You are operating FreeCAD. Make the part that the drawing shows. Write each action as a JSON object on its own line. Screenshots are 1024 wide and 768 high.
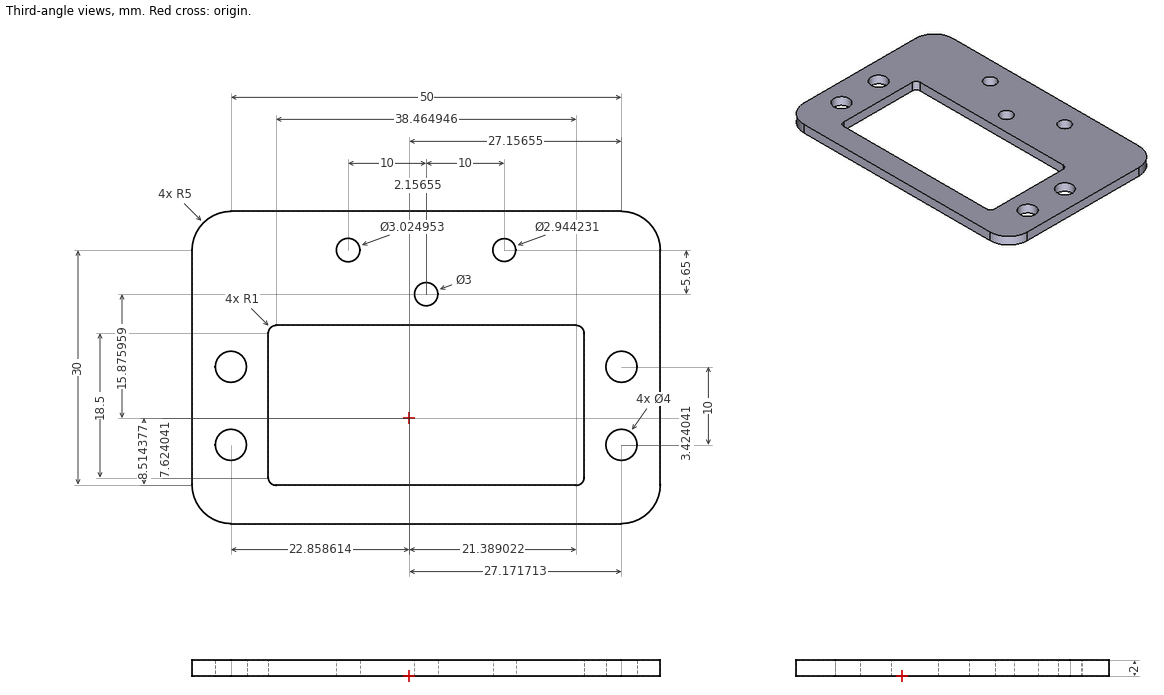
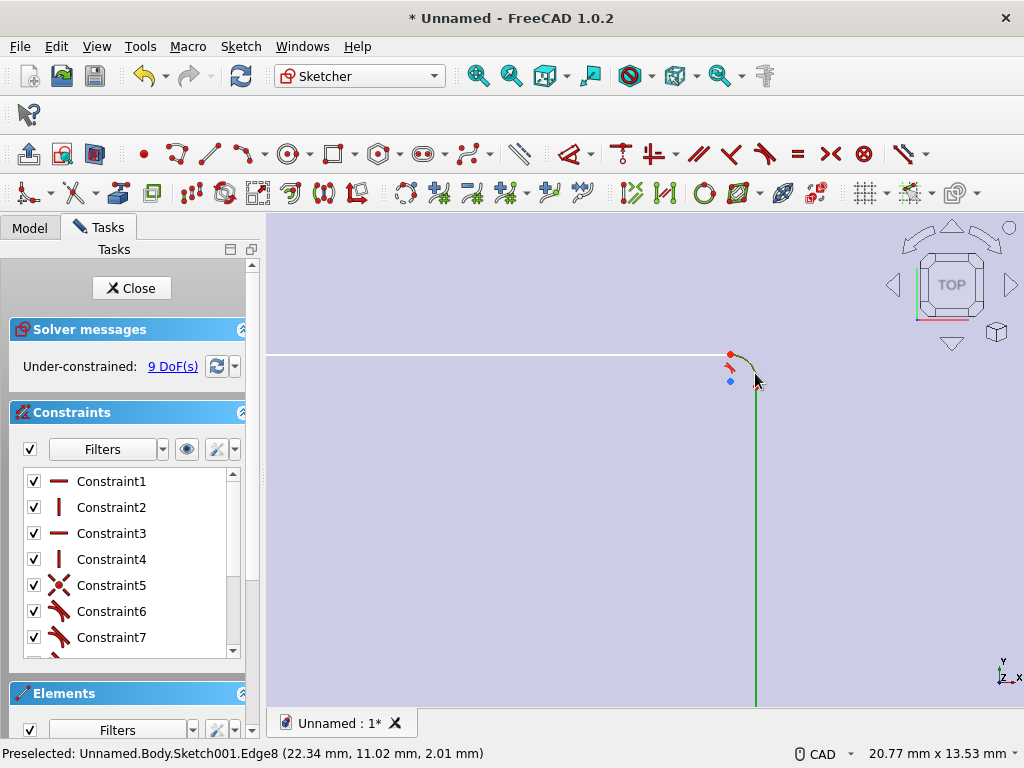
{"action": "key", "text": "t"}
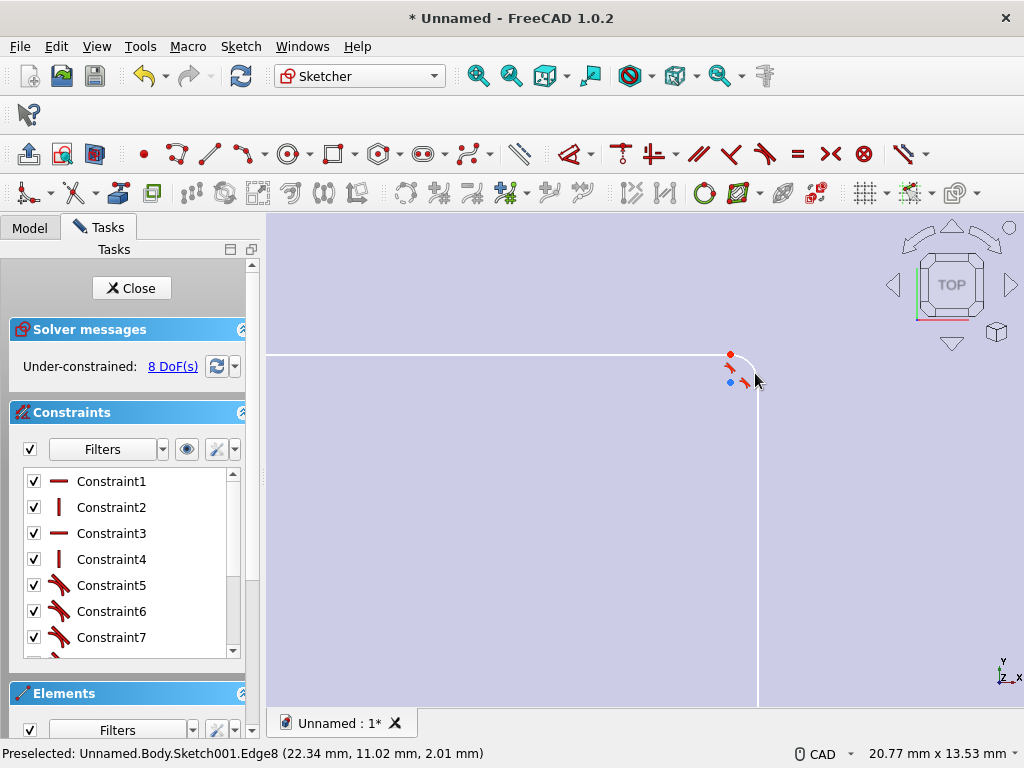
{"action": "scroll", "coordinate": [759, 375], "scroll_direction": "down", "scroll_amount": 7}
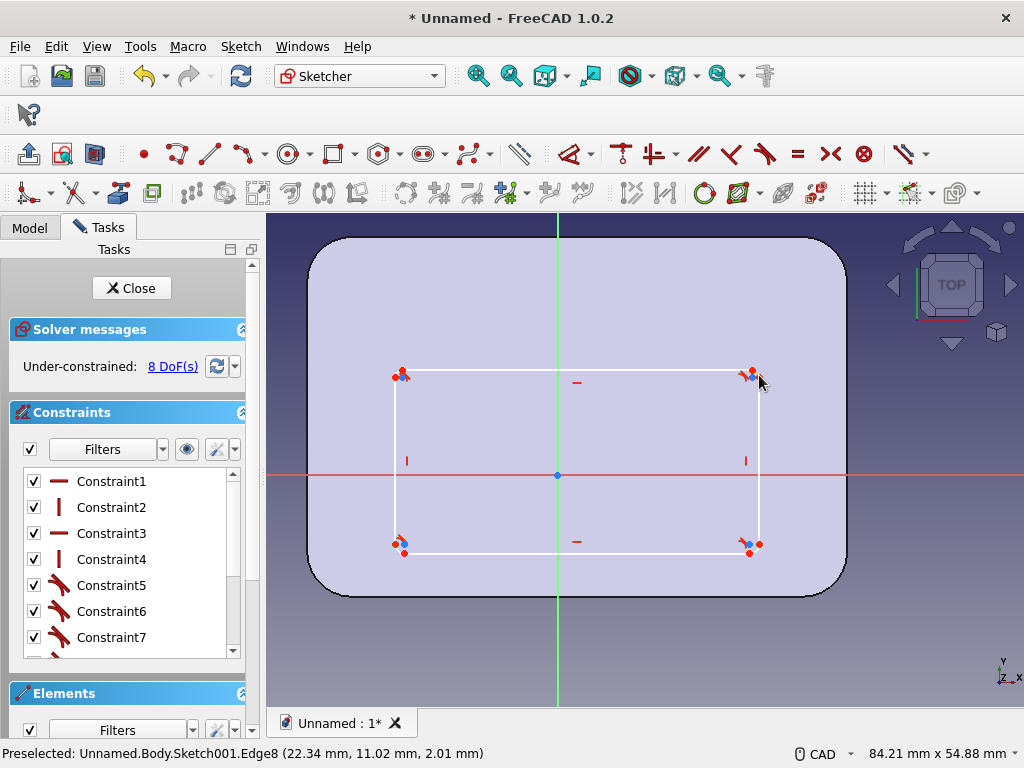
{"action": "scroll", "coordinate": [399, 371], "scroll_direction": "up", "scroll_amount": 7}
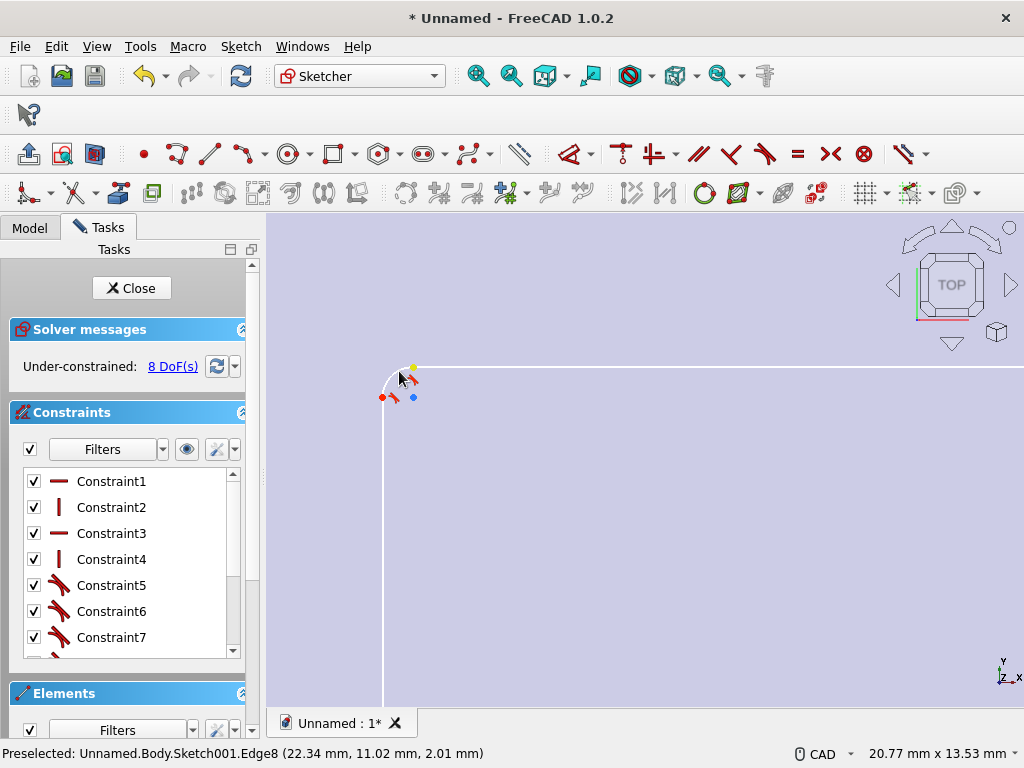
{"action": "left_click", "coordinate": [399, 370]}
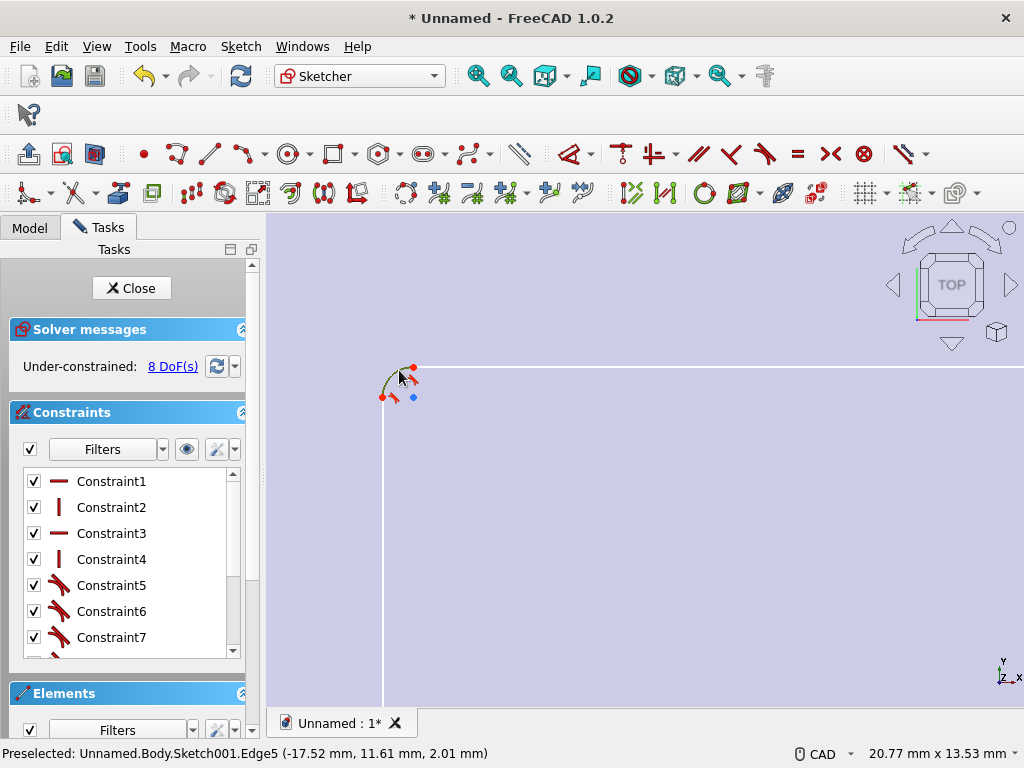
{"action": "scroll", "coordinate": [398, 371], "scroll_direction": "down", "scroll_amount": 7}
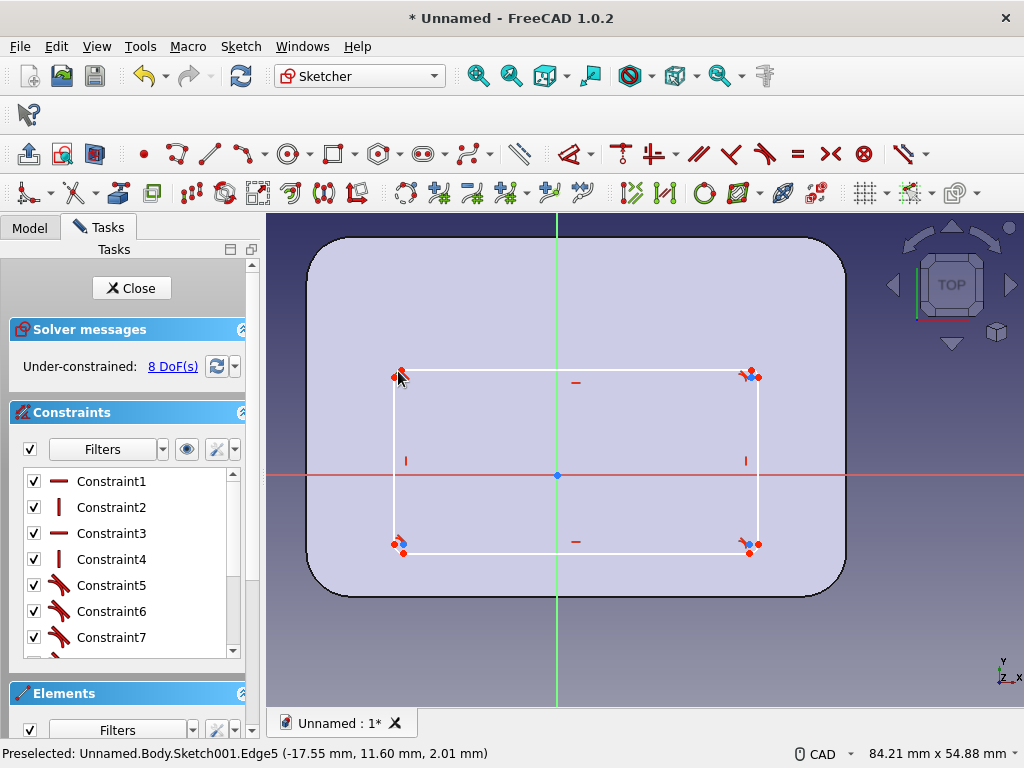
{"action": "scroll", "coordinate": [395, 548], "scroll_direction": "up", "scroll_amount": 6}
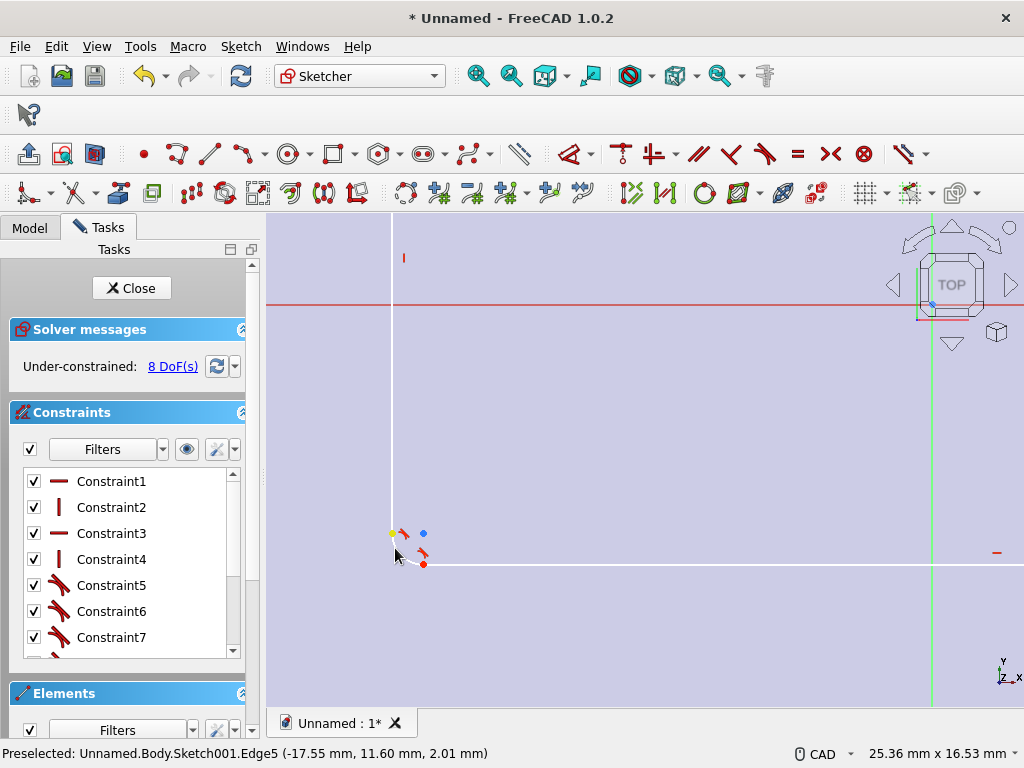
{"action": "left_click", "coordinate": [396, 548]}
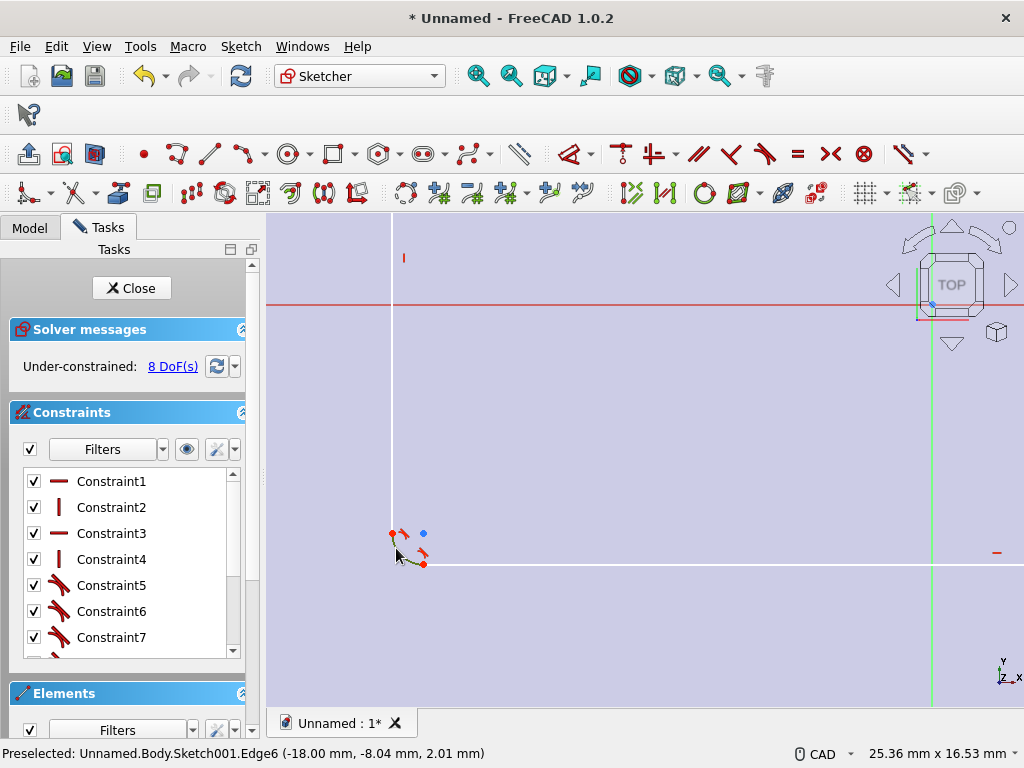
{"action": "scroll", "coordinate": [395, 548], "scroll_direction": "down", "scroll_amount": 6}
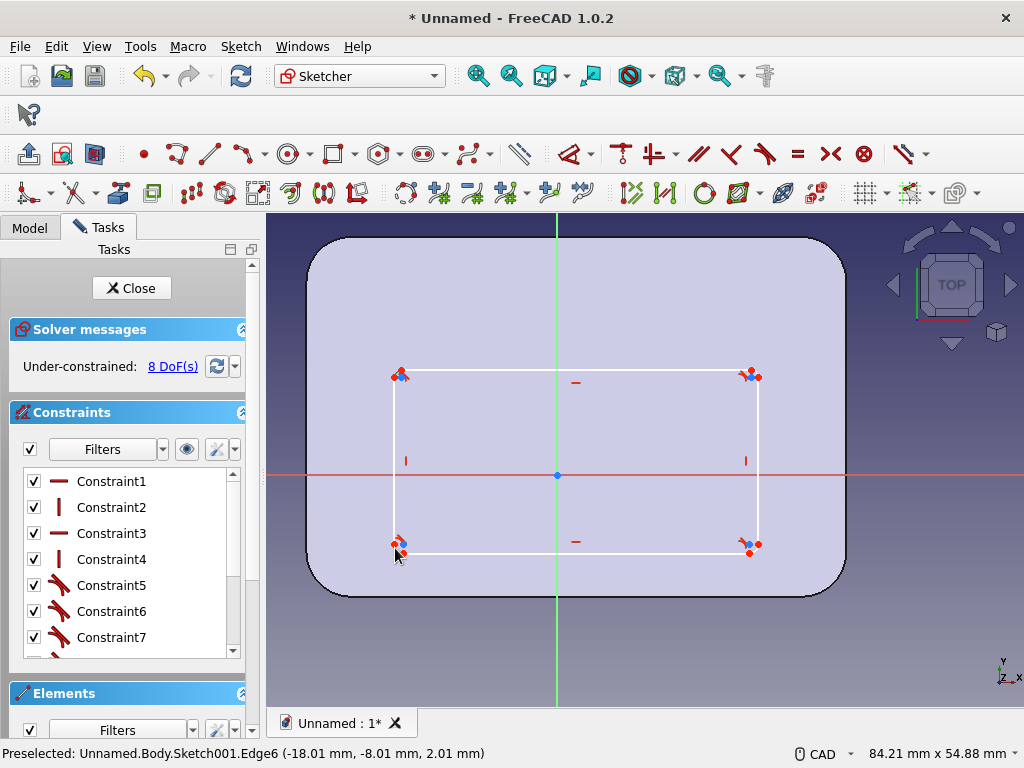
{"action": "scroll", "coordinate": [753, 553], "scroll_direction": "up", "scroll_amount": 6}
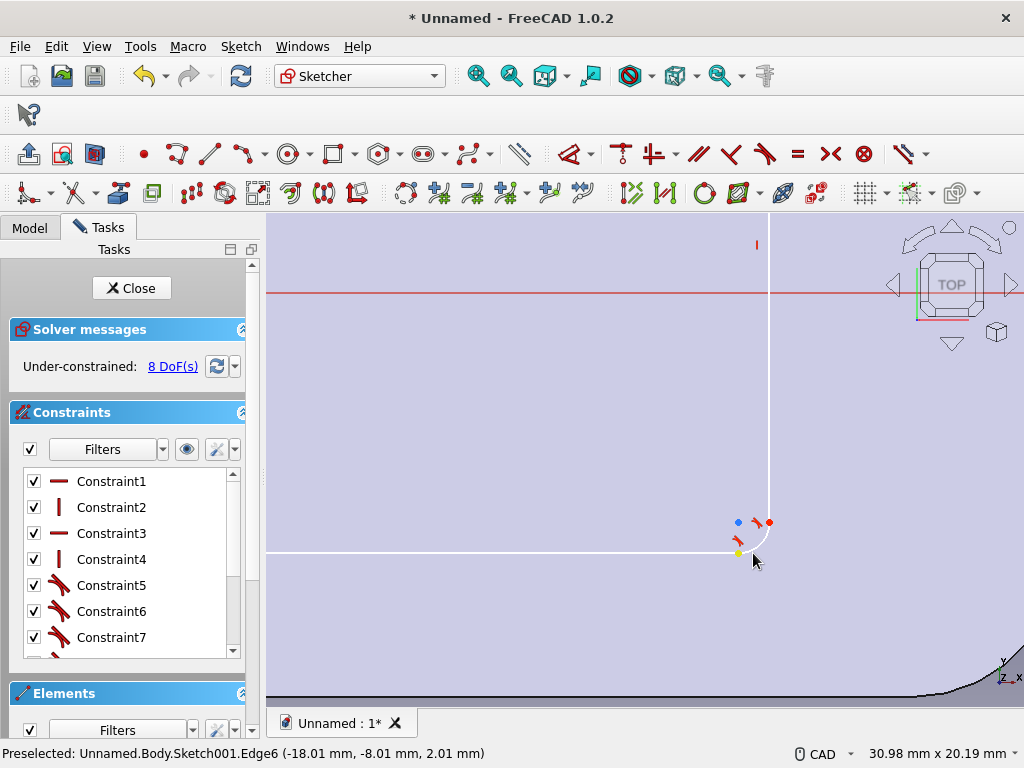
{"action": "left_click", "coordinate": [753, 550]}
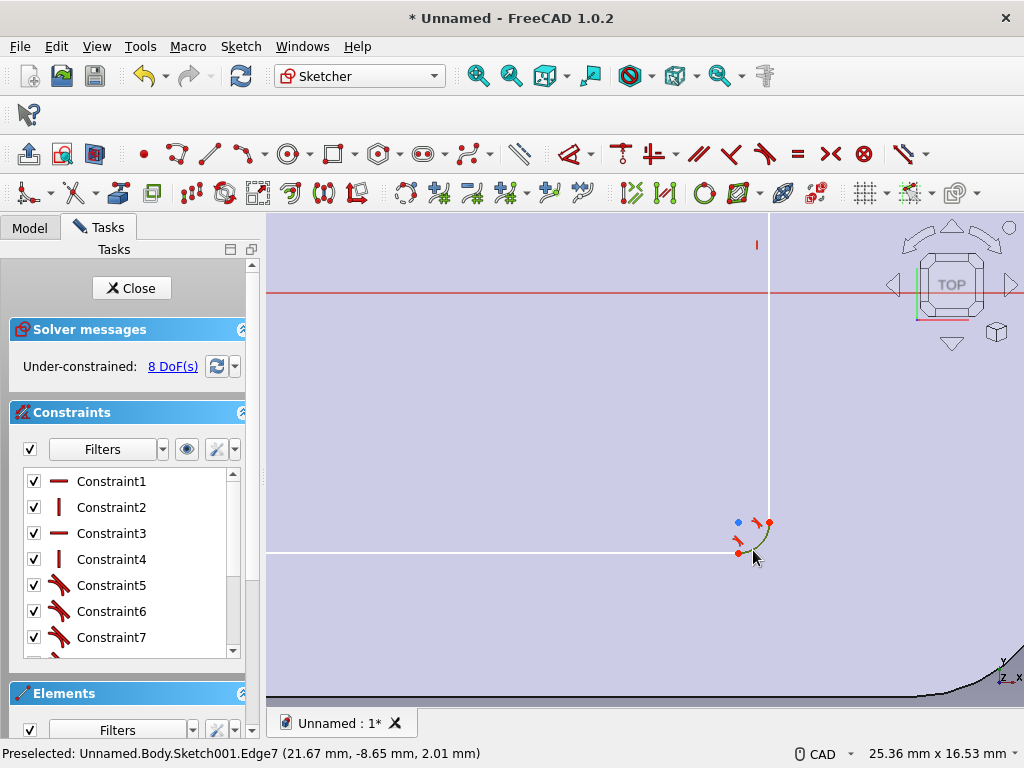
{"action": "scroll", "coordinate": [754, 553], "scroll_direction": "down", "scroll_amount": 6}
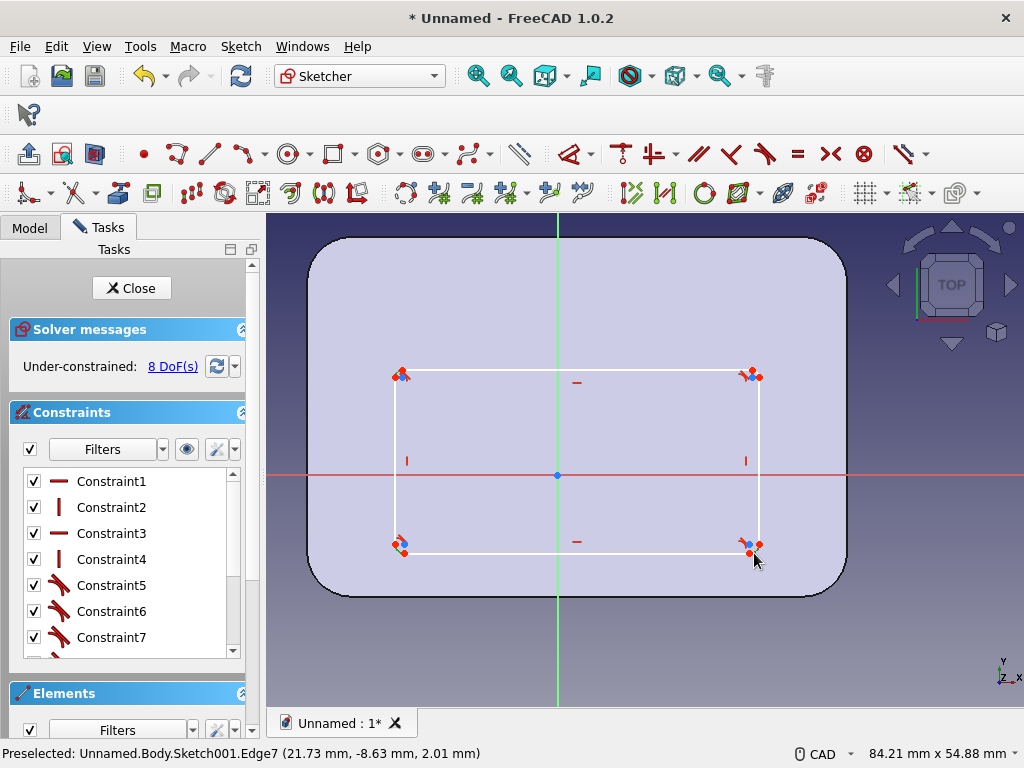
{"action": "scroll", "coordinate": [758, 374], "scroll_direction": "up", "scroll_amount": 8}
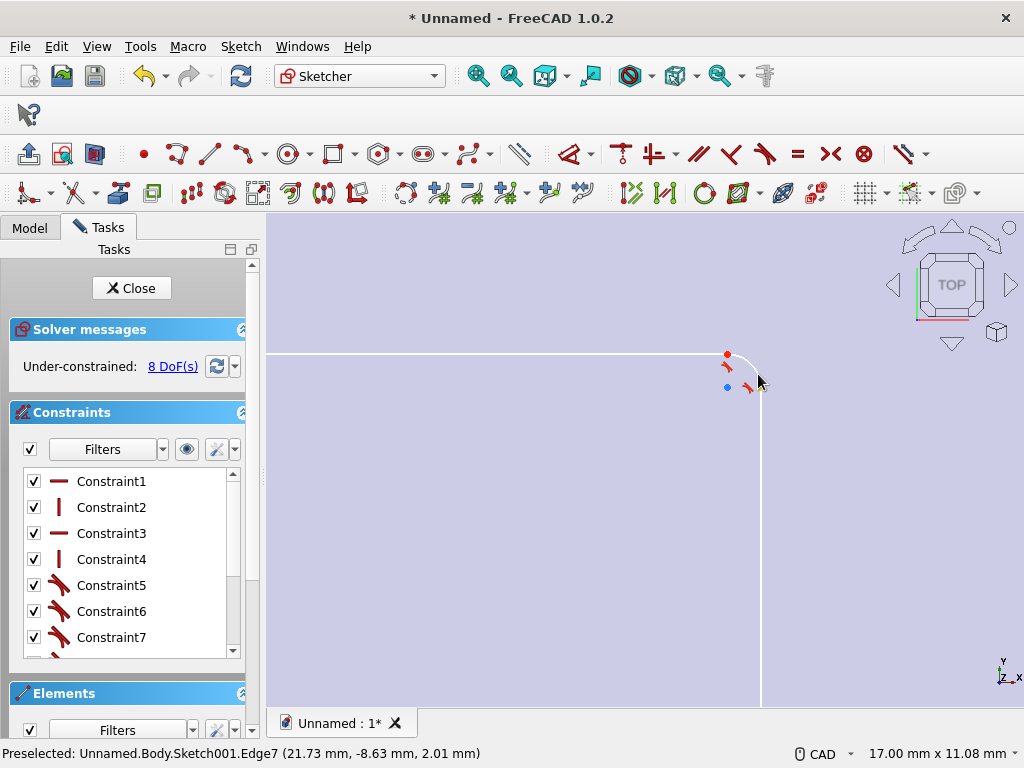
{"action": "left_click", "coordinate": [757, 373]}